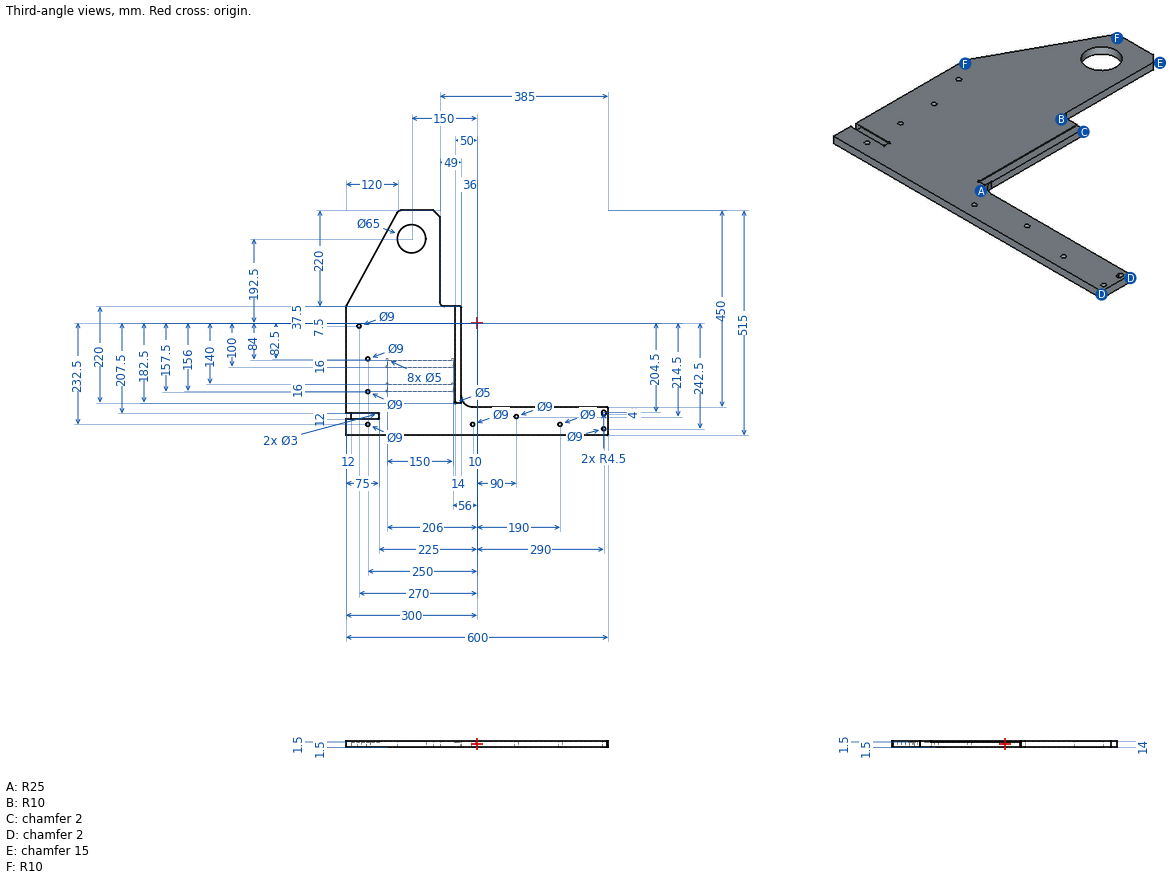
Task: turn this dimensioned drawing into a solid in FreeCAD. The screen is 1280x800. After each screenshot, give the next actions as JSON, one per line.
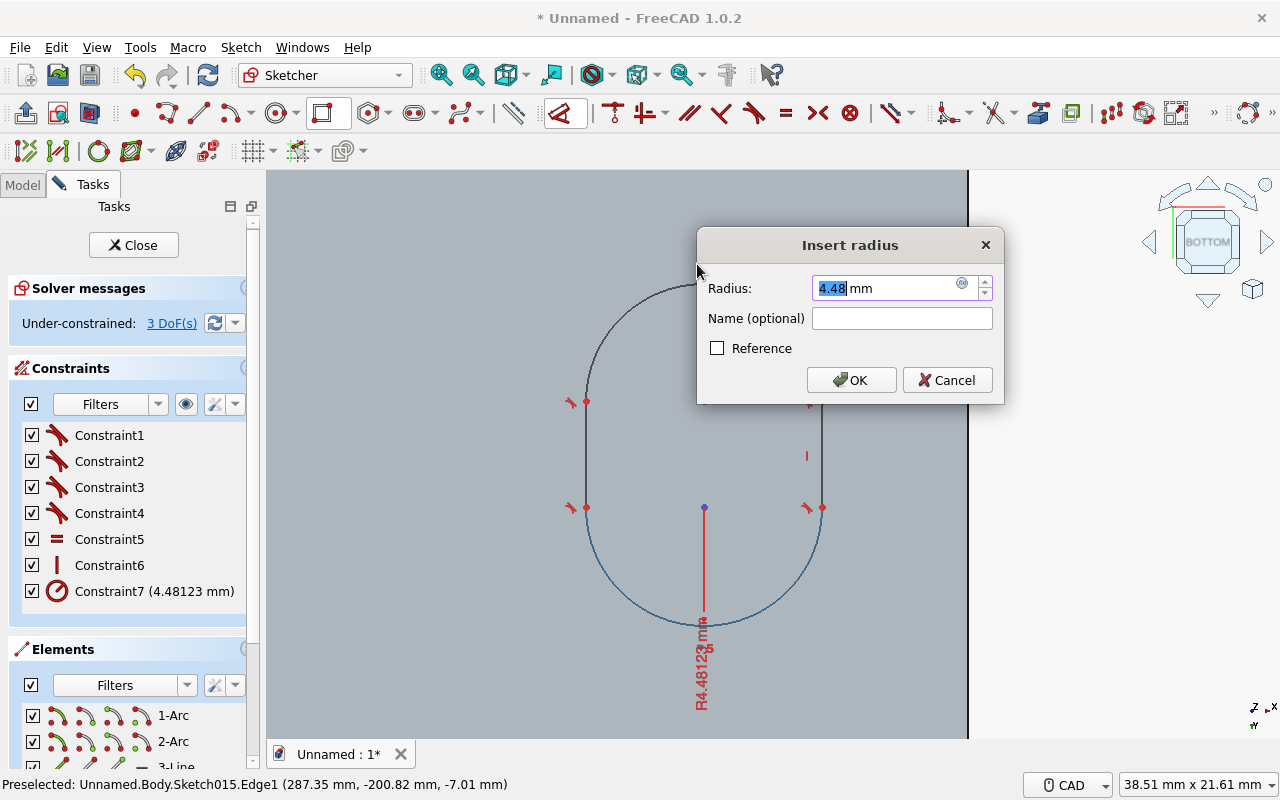
{"action": "type", "text": "4.5"}
{"action": "key", "text": "Return"}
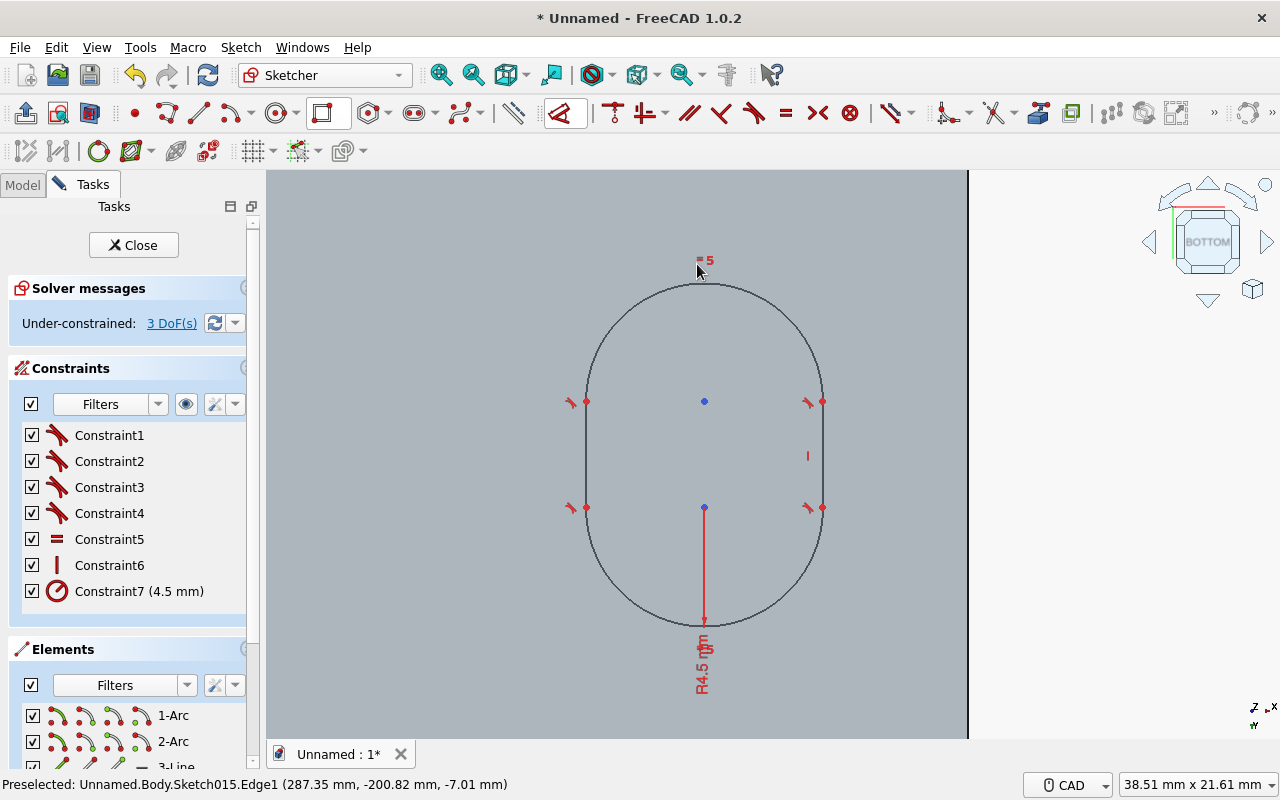
{"action": "left_click", "coordinate": [586, 476]}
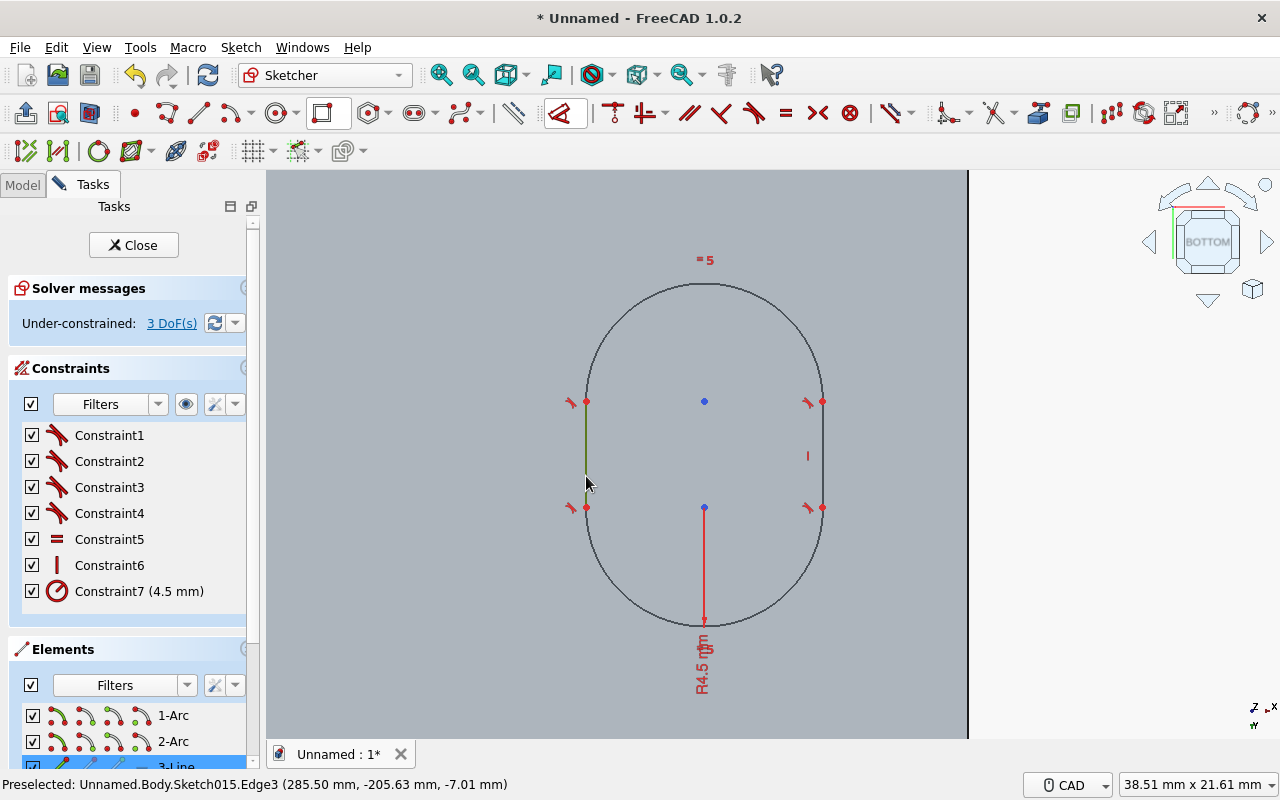
{"action": "left_click", "coordinate": [582, 114]}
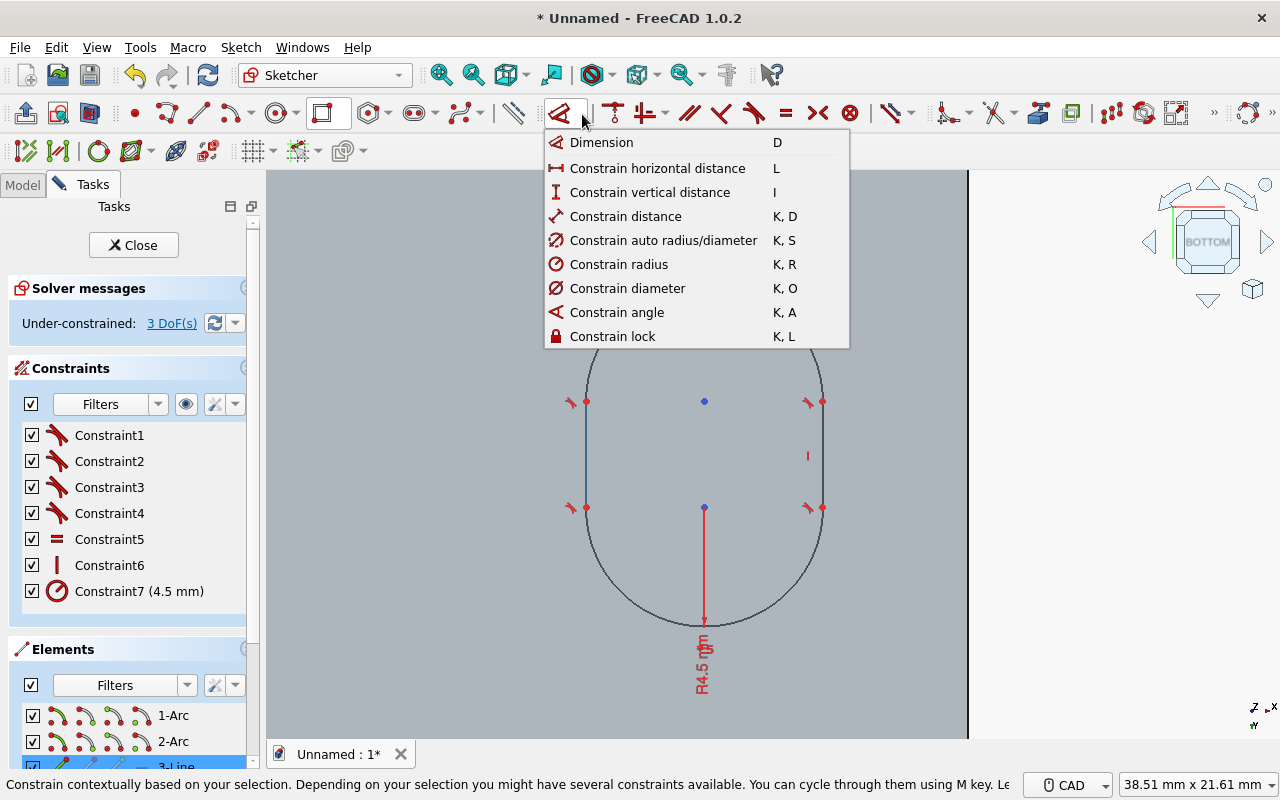
{"action": "left_click", "coordinate": [697, 192]}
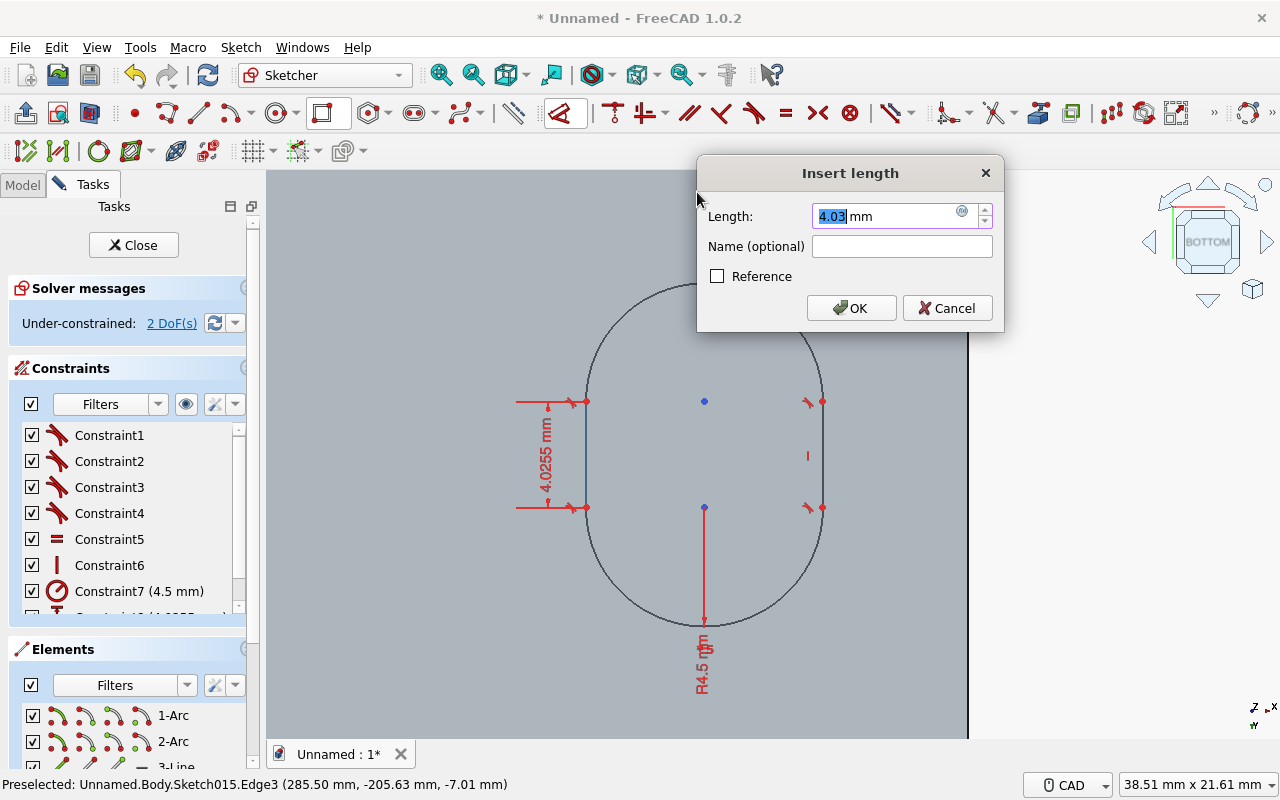
{"action": "type", "text": "4"}
{"action": "key", "text": "Return"}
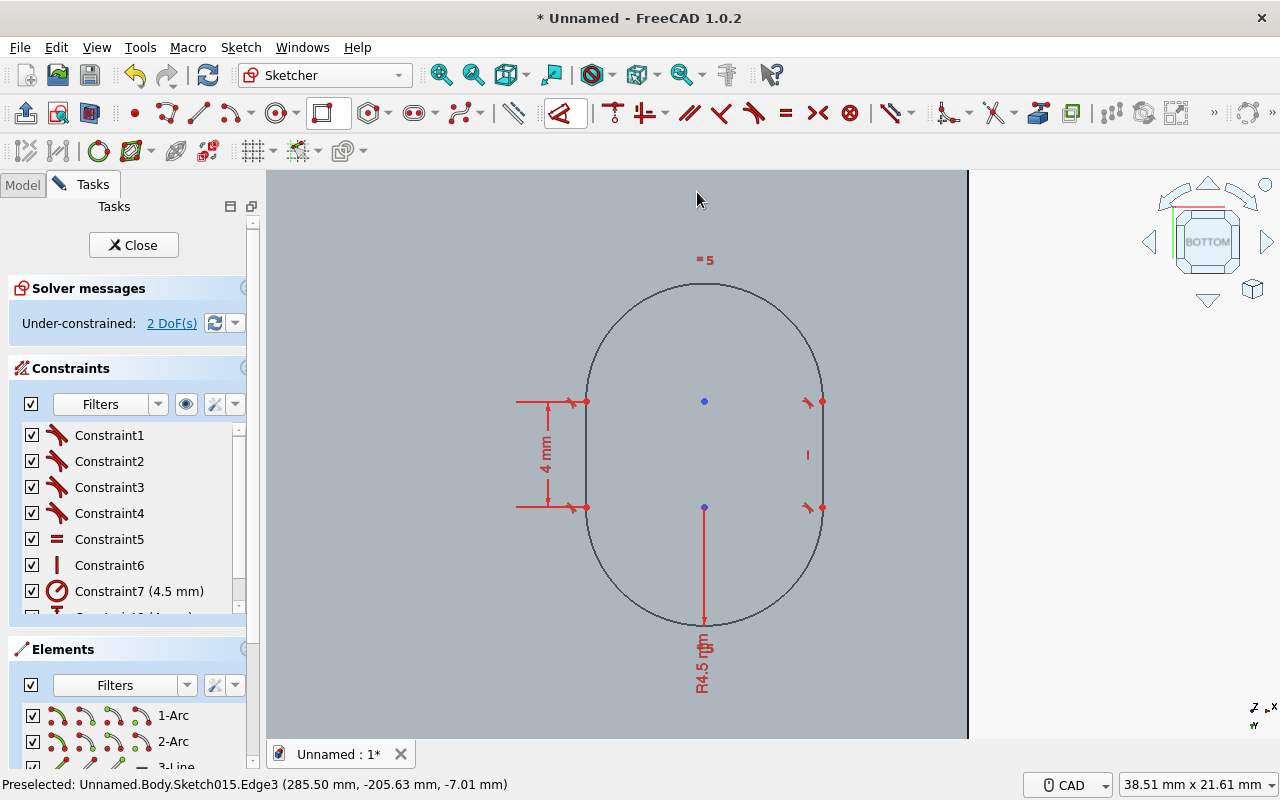
{"action": "left_click", "coordinate": [704, 507]}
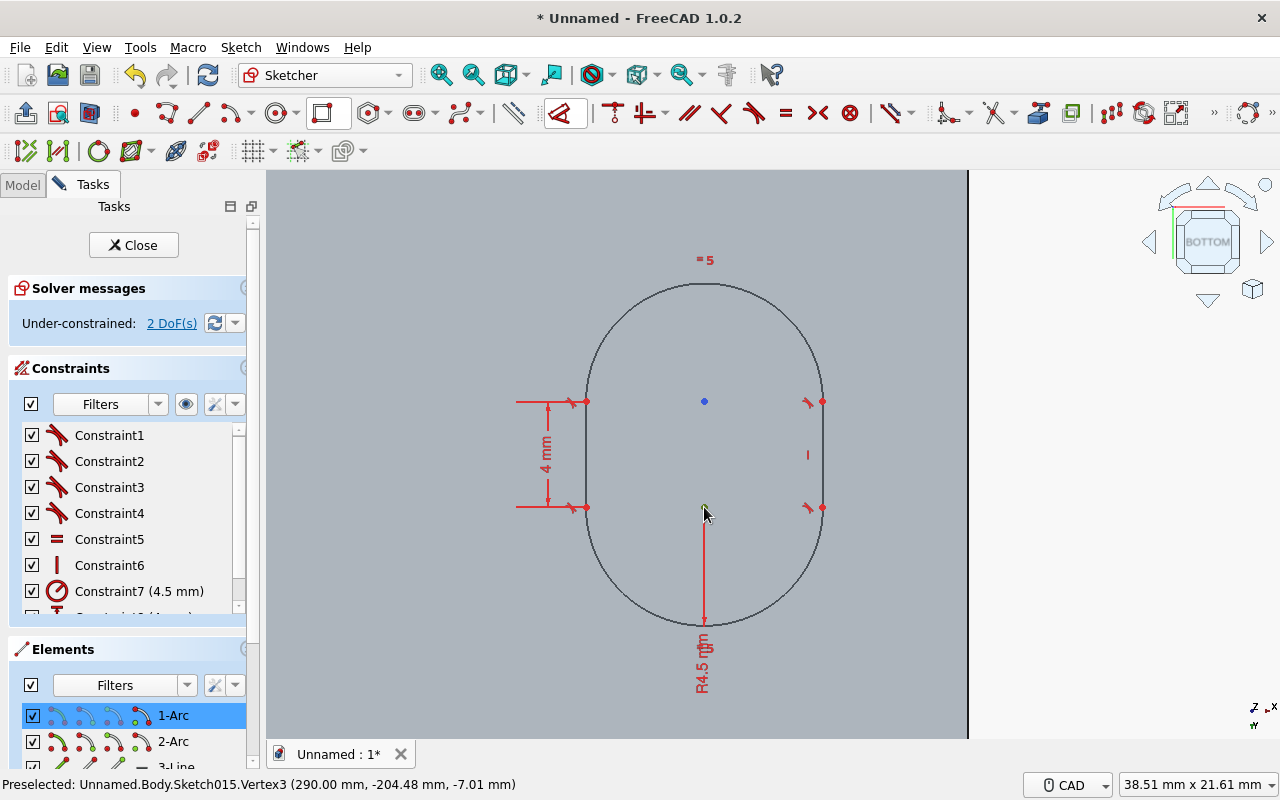
{"action": "key", "text": "l"}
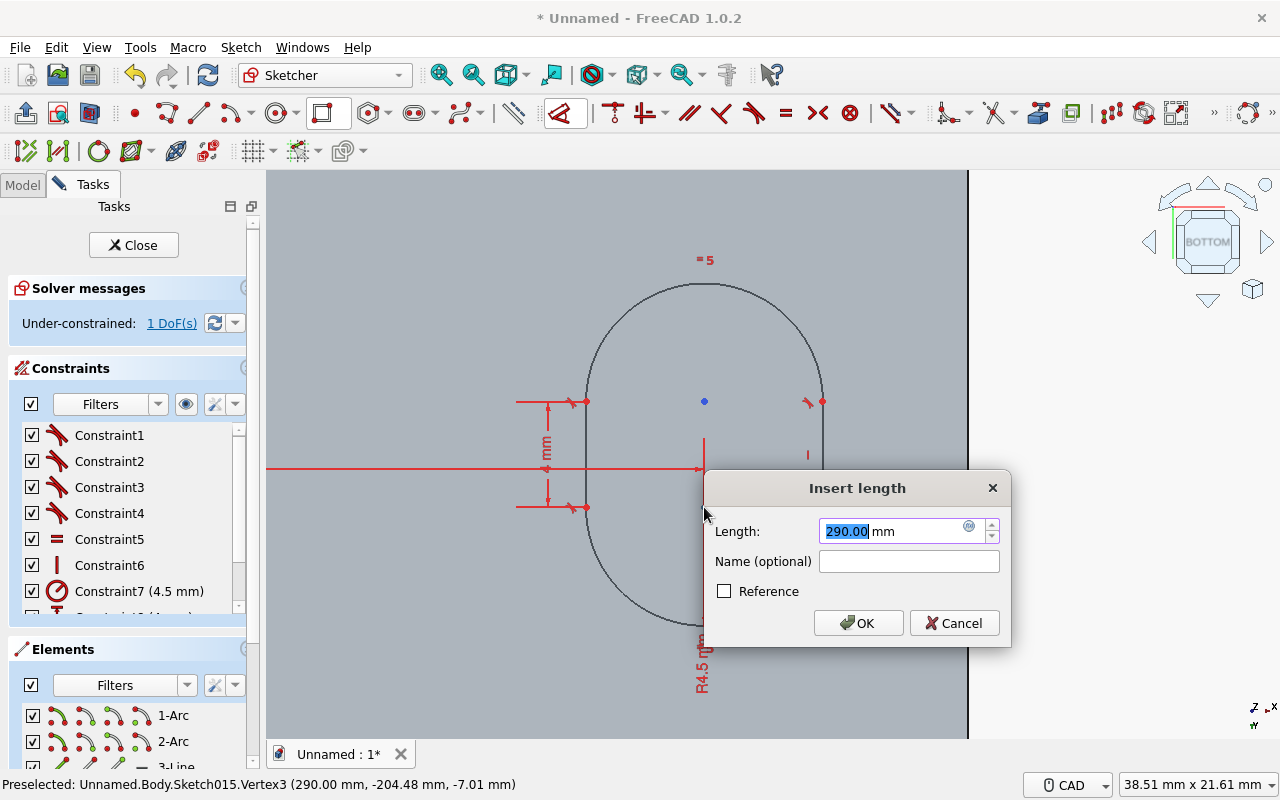
{"action": "type", "text": "290"}
{"action": "key", "text": "Return"}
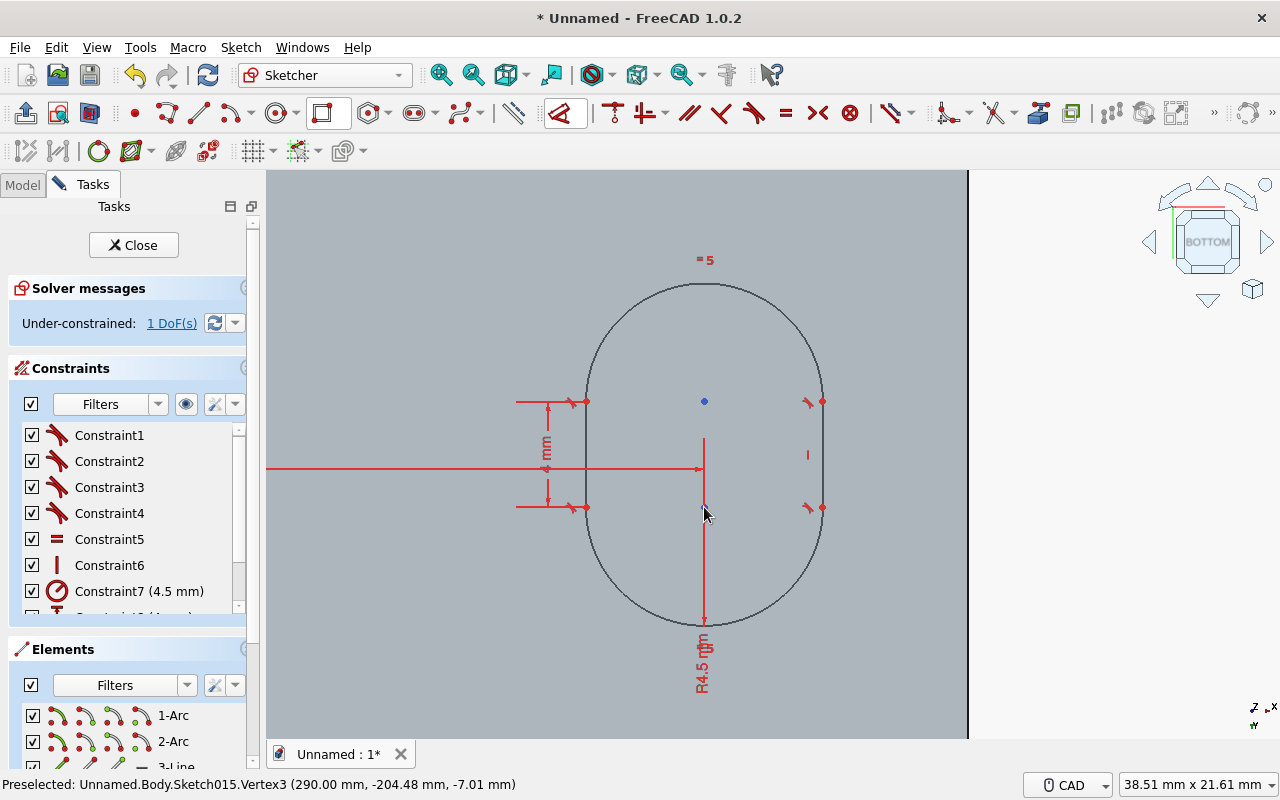
{"action": "left_click", "coordinate": [586, 507]}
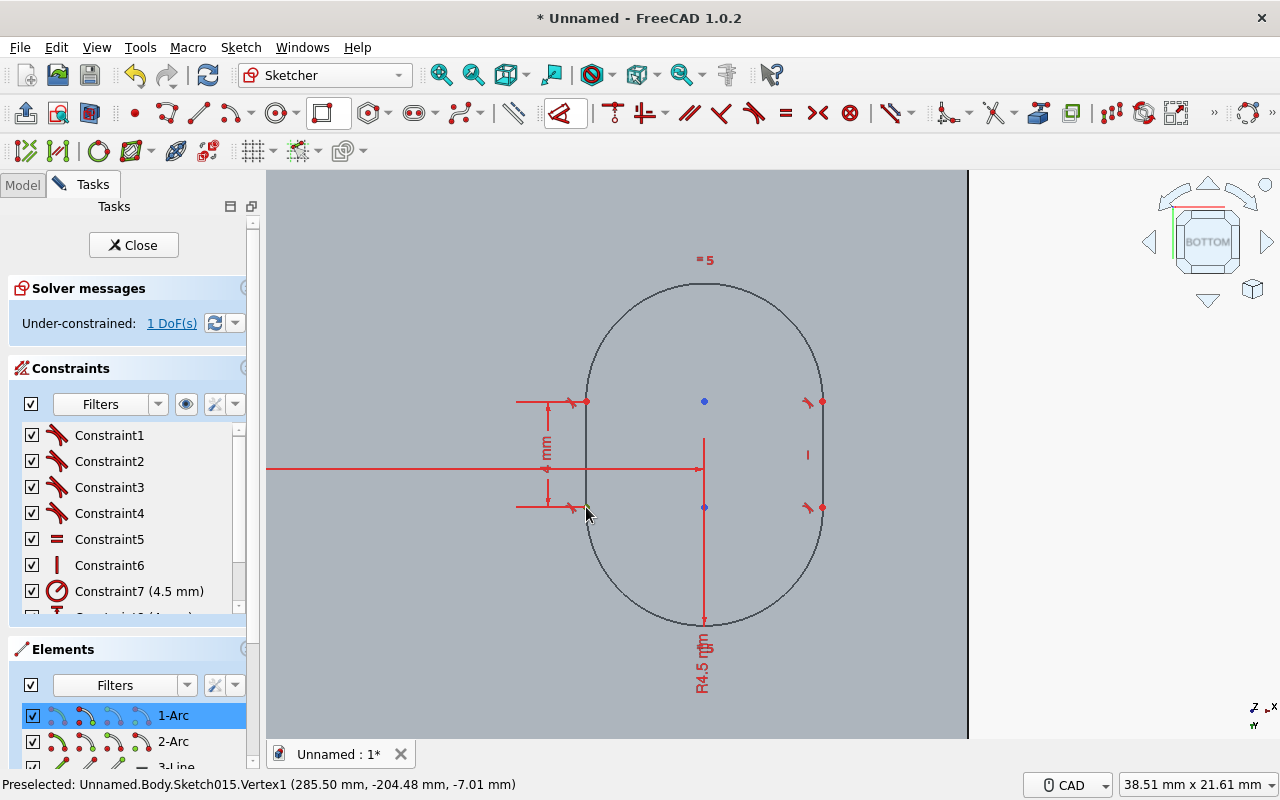
{"action": "left_click", "coordinate": [582, 114]}